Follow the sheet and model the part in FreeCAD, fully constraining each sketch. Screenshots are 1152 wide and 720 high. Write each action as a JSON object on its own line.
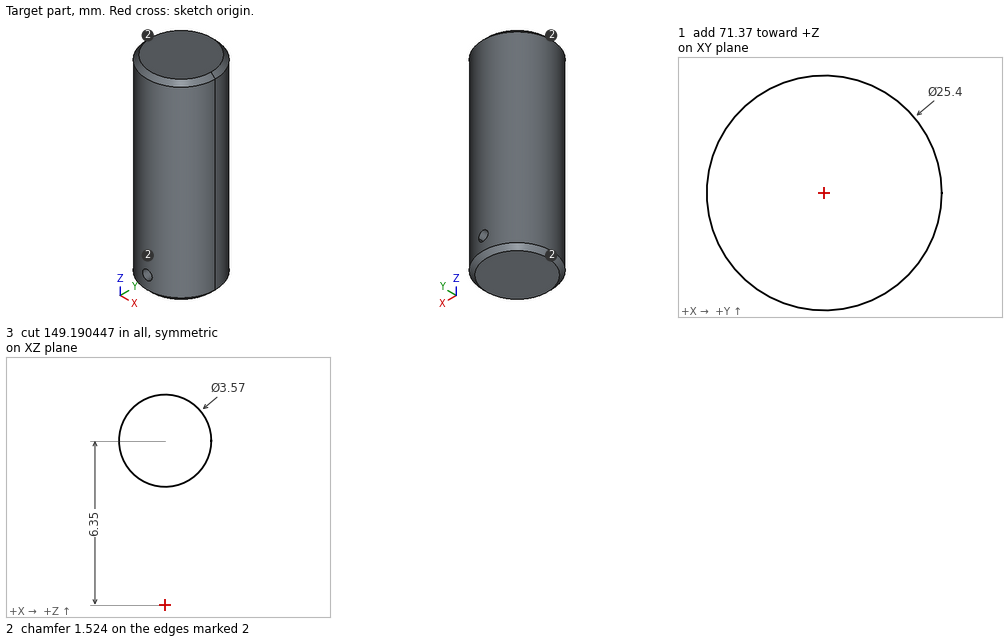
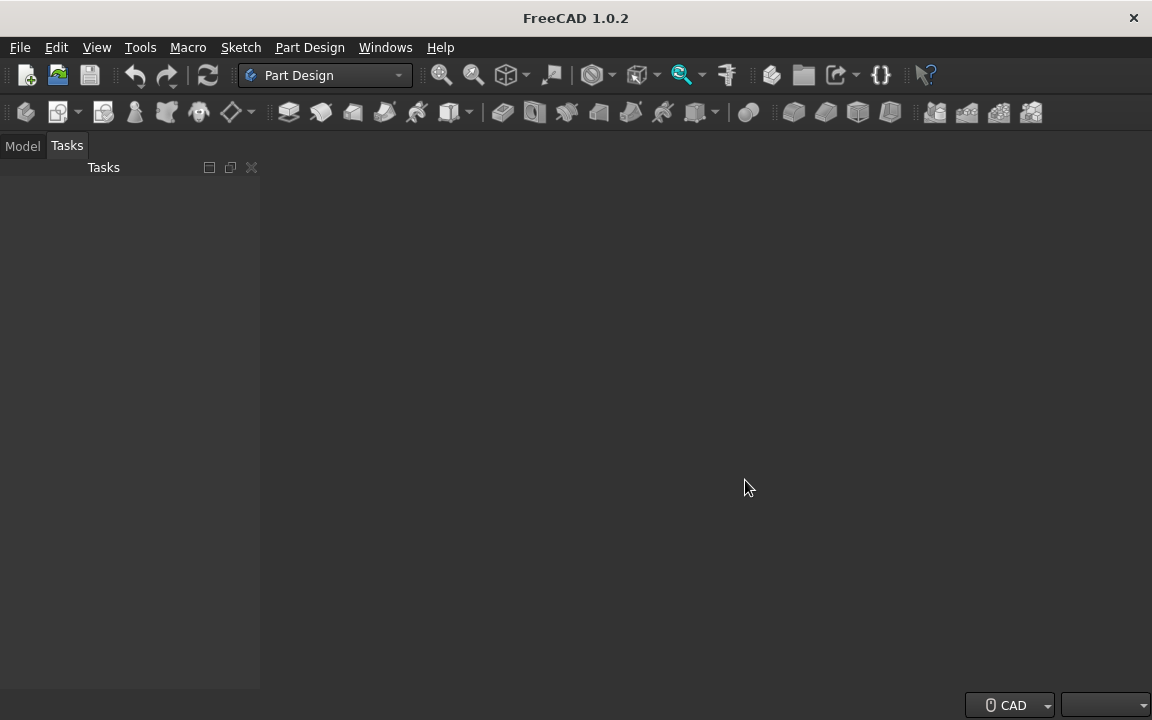
{"action": "left_click", "coordinate": [26, 76]}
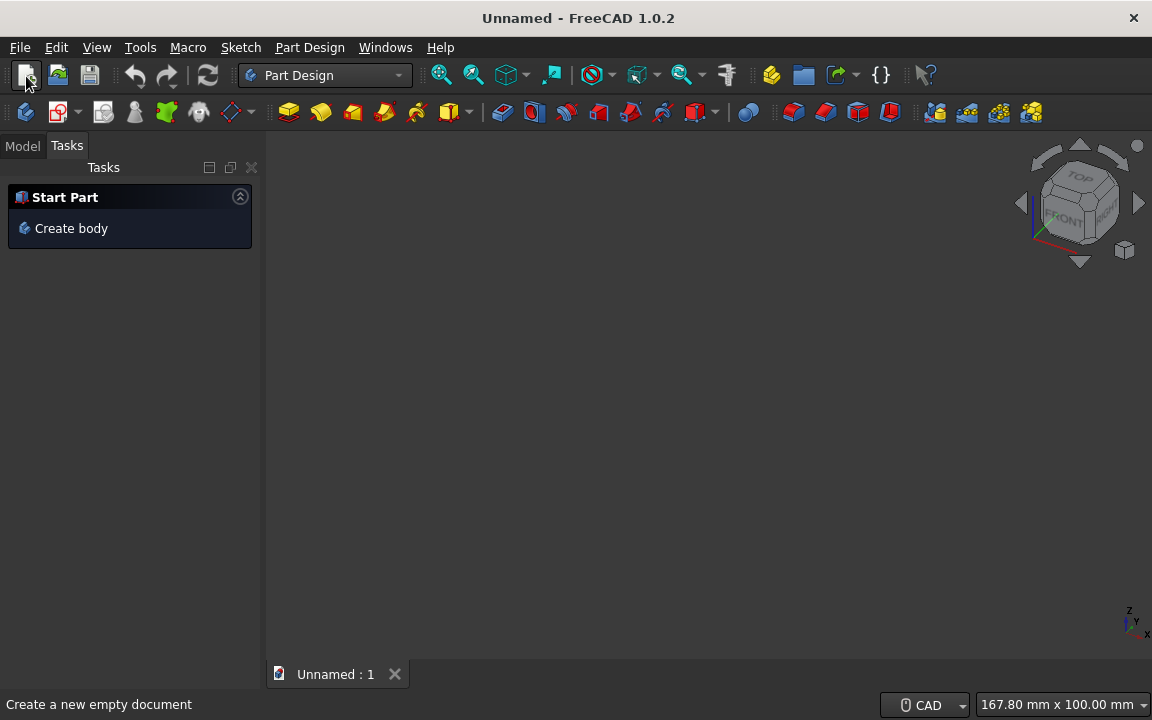
{"action": "left_click", "coordinate": [58, 112]}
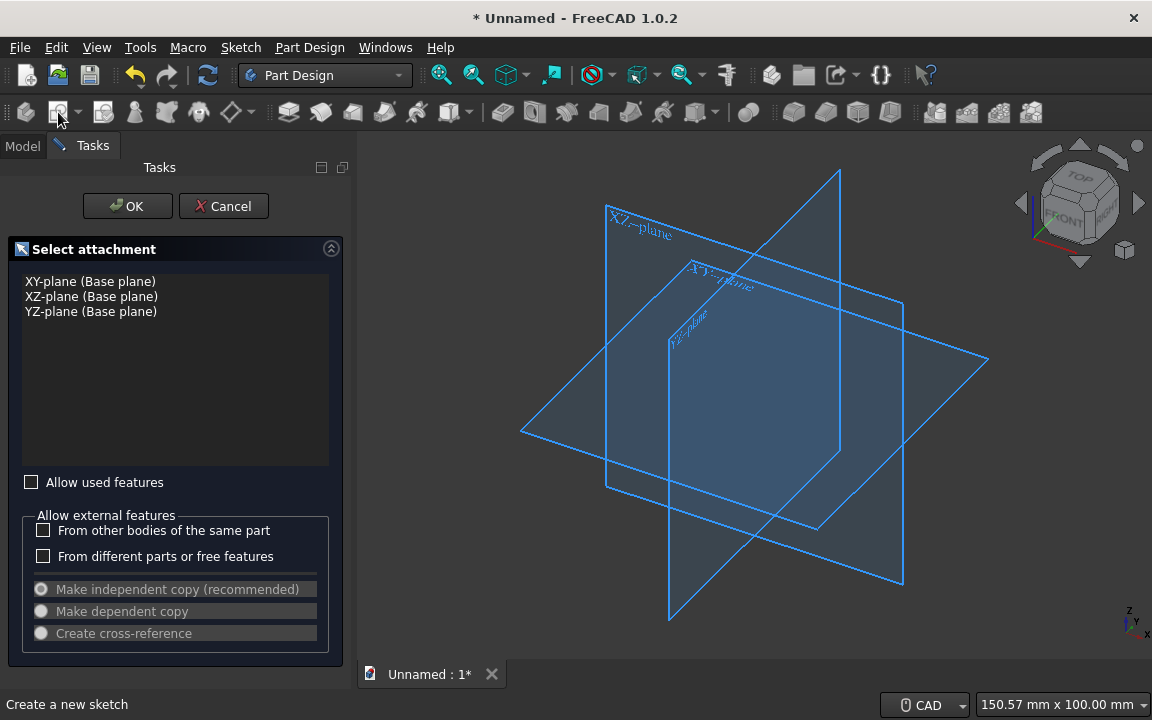
{"action": "left_click", "coordinate": [82, 282]}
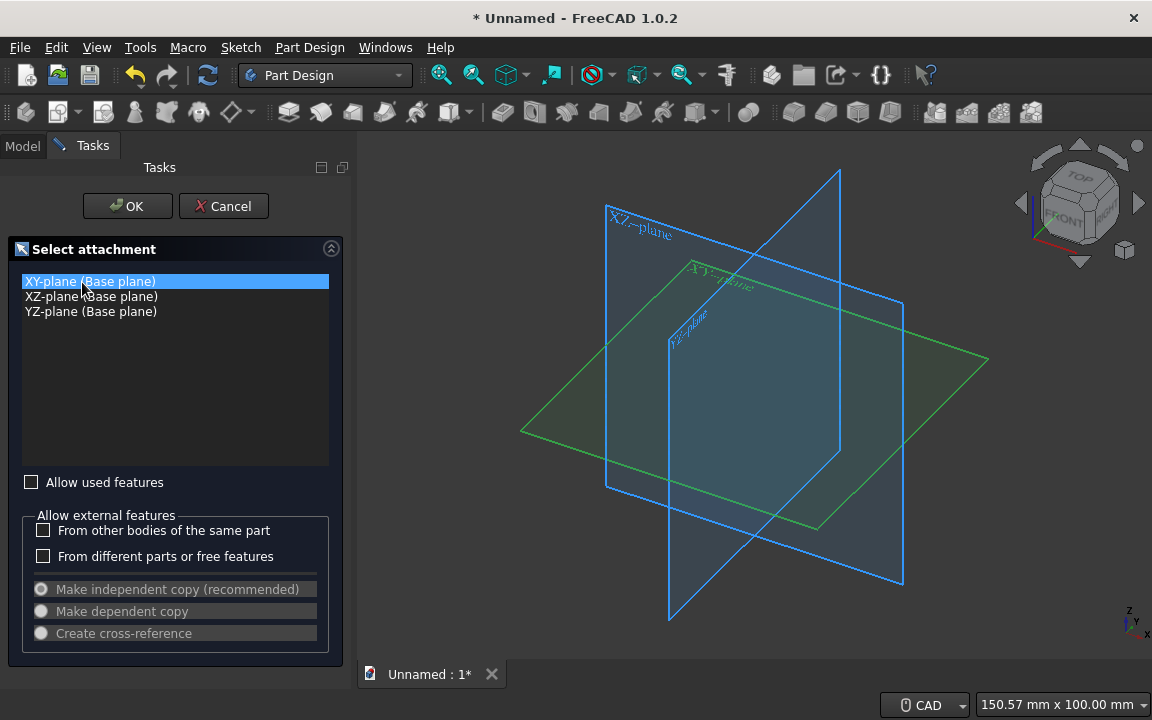
{"action": "left_click", "coordinate": [128, 206]}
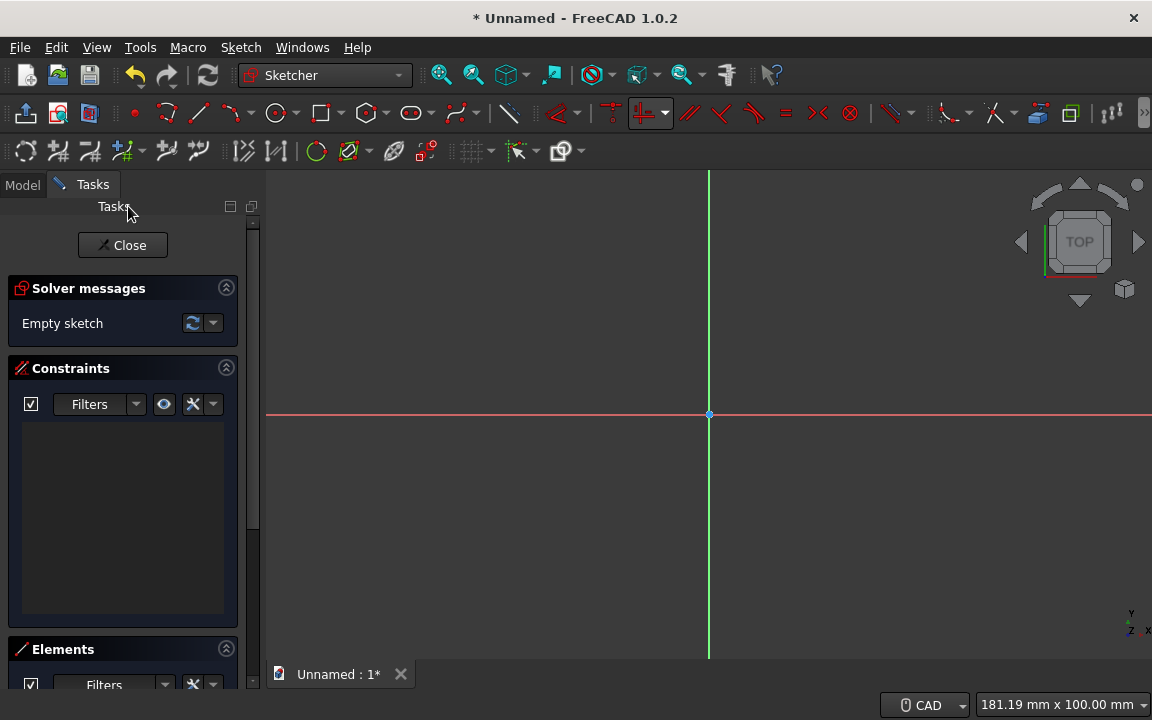
{"action": "scroll", "coordinate": [749, 415], "scroll_direction": "up", "scroll_amount": 5}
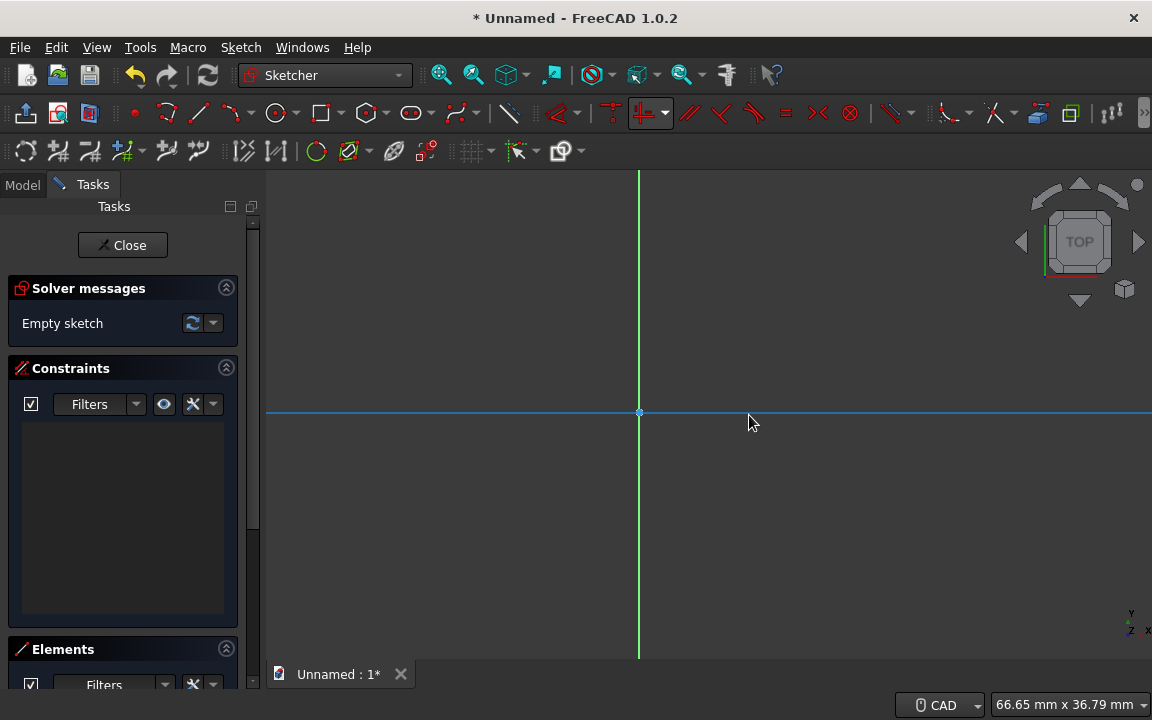
{"action": "left_click", "coordinate": [276, 114]}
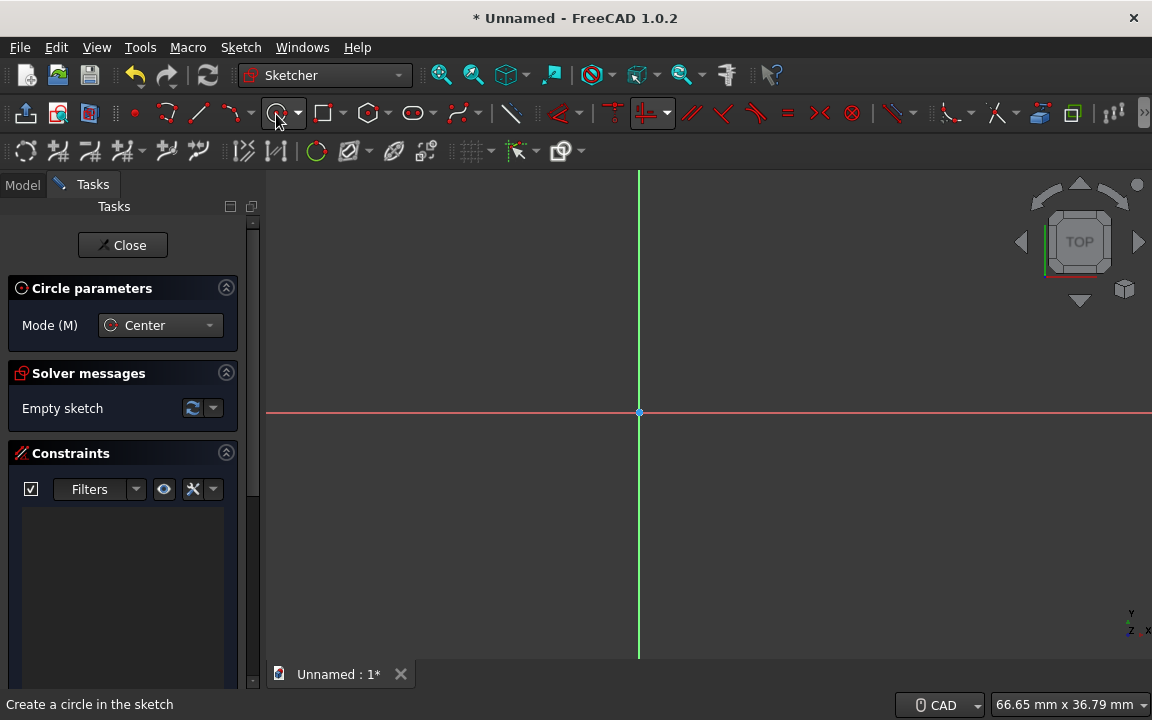
{"action": "left_click", "coordinate": [639, 413]}
{"action": "left_click", "coordinate": [759, 293]}
{"action": "key", "text": "Escape"}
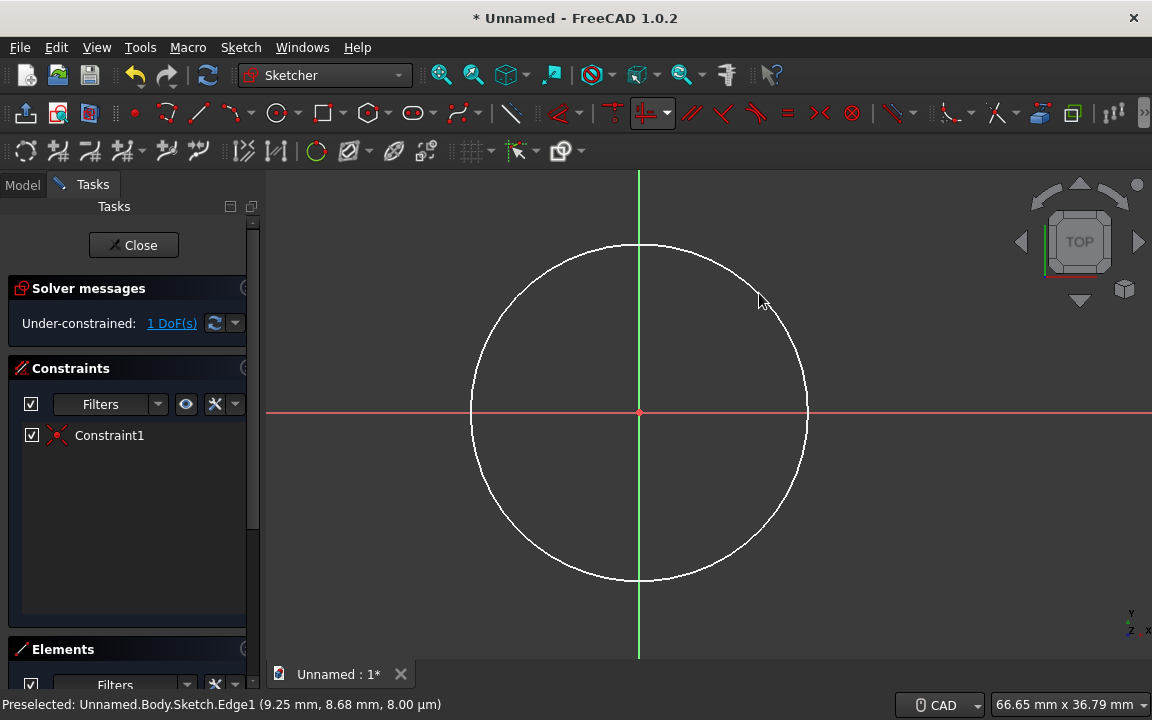
{"action": "left_click", "coordinate": [558, 114]}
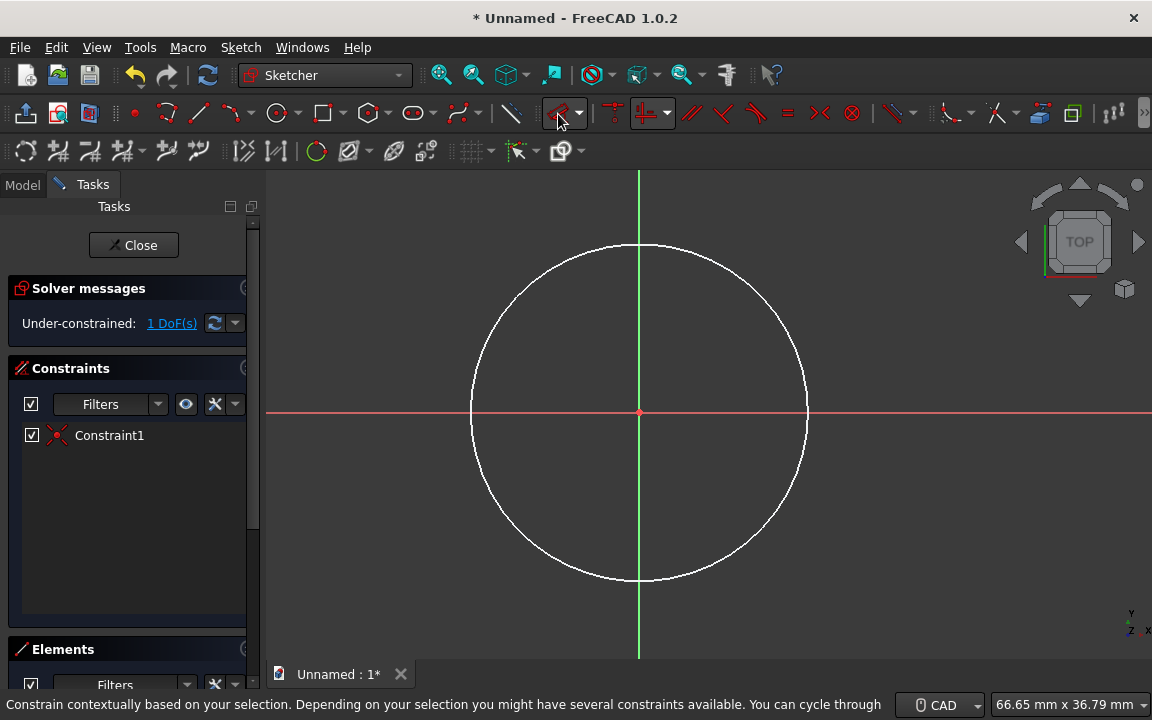
{"action": "left_click", "coordinate": [758, 293]}
{"action": "left_click", "coordinate": [781, 270]}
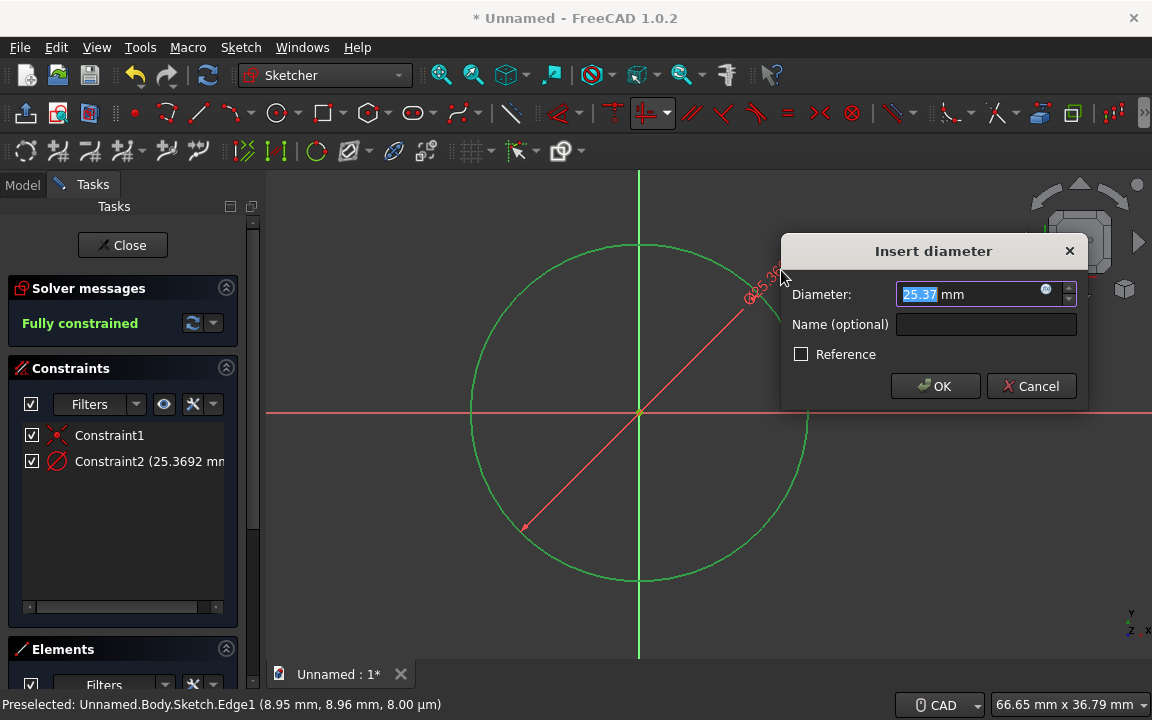
{"action": "type", "text": "25.4"}
{"action": "key", "text": "Return"}
{"action": "key", "text": "Escape"}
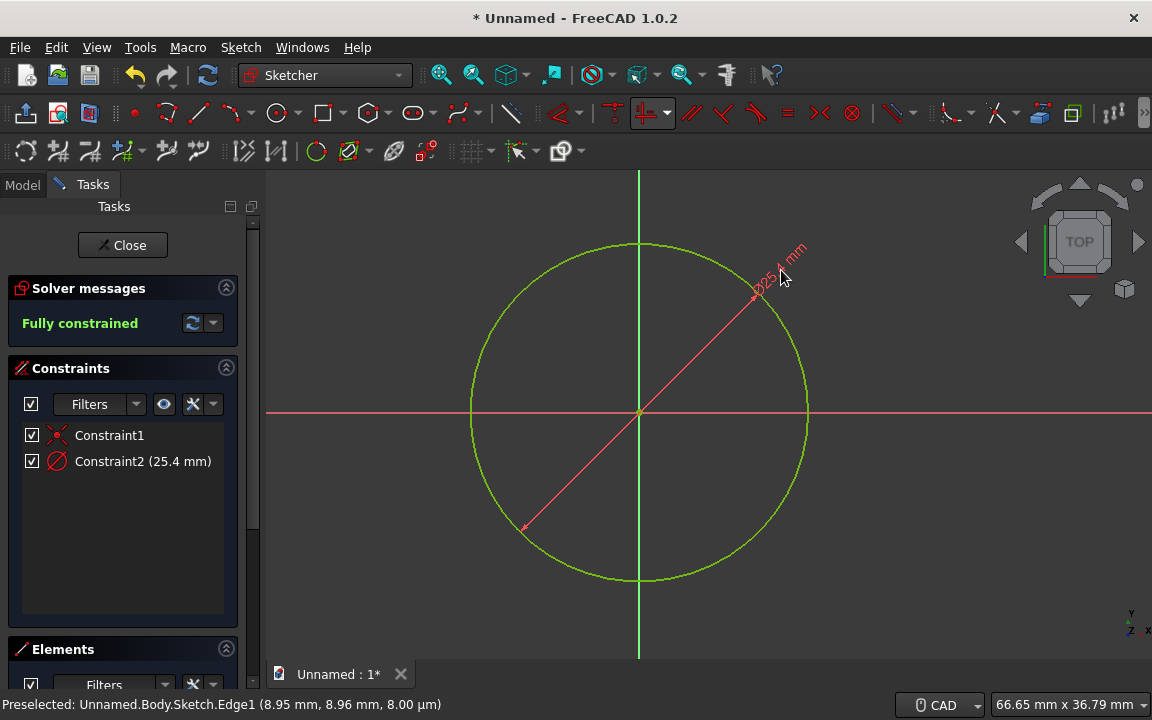
{"action": "left_click", "coordinate": [123, 245]}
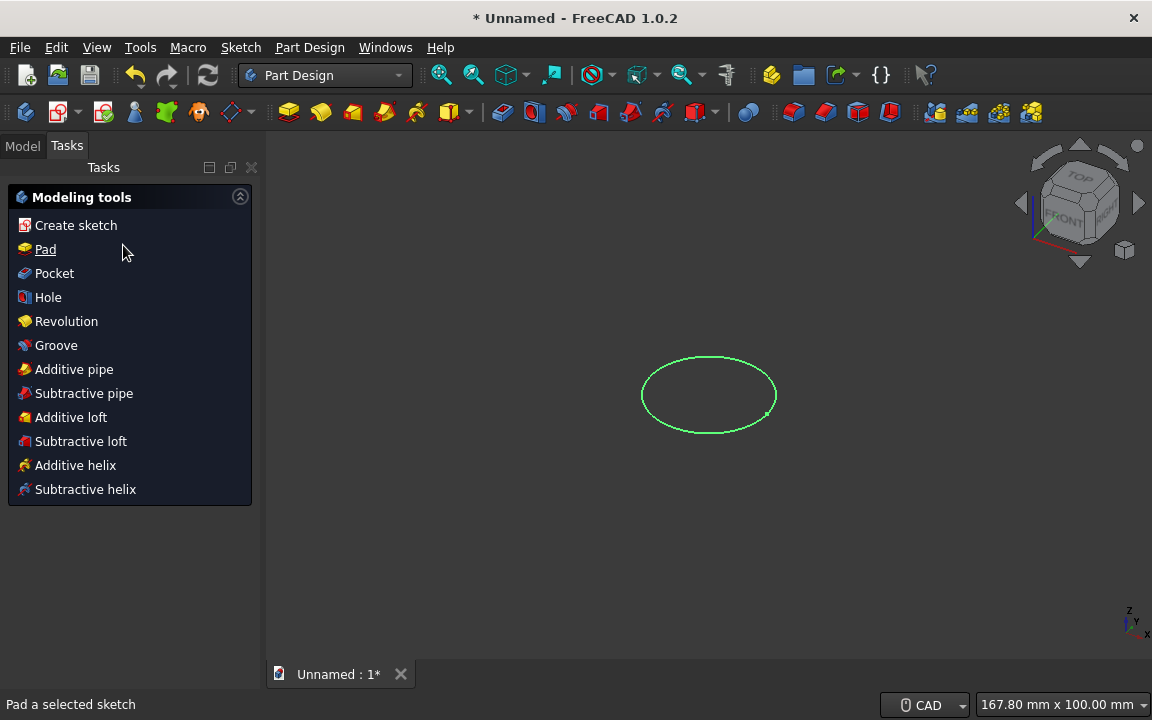
{"action": "left_click", "coordinate": [290, 112]}